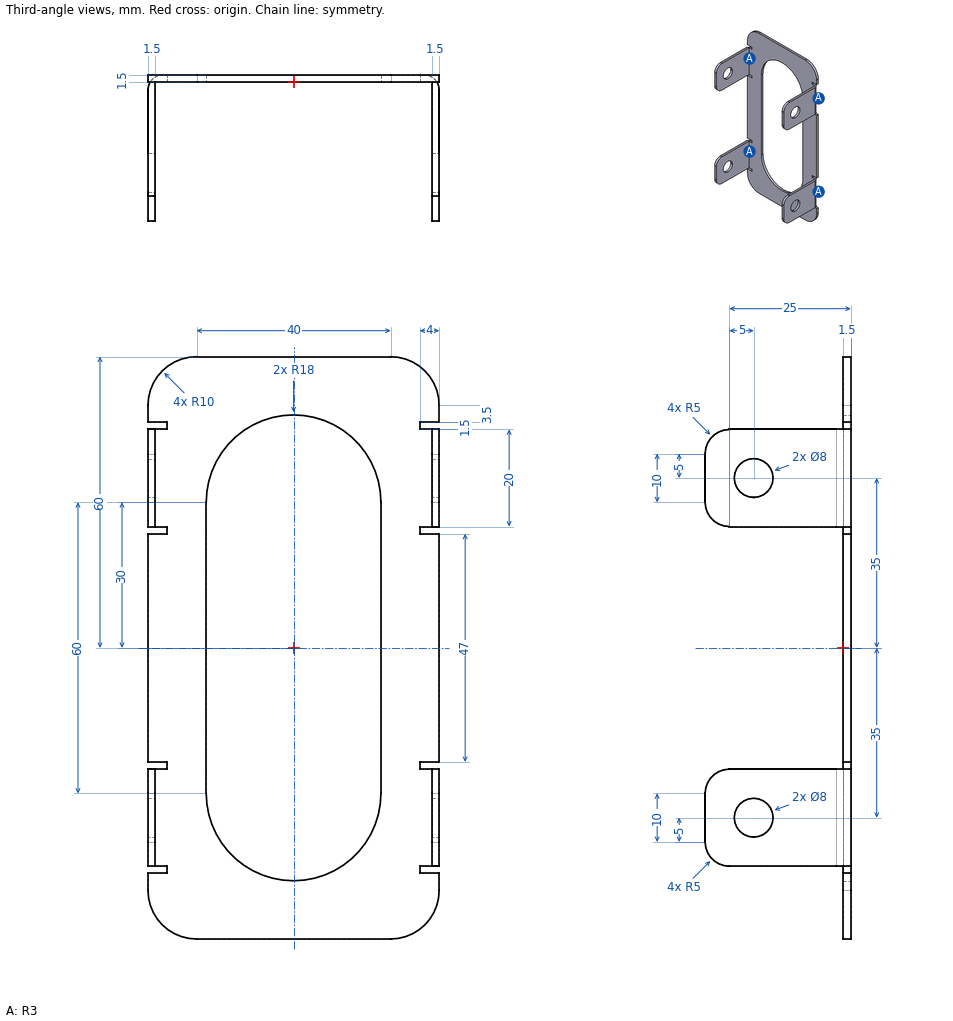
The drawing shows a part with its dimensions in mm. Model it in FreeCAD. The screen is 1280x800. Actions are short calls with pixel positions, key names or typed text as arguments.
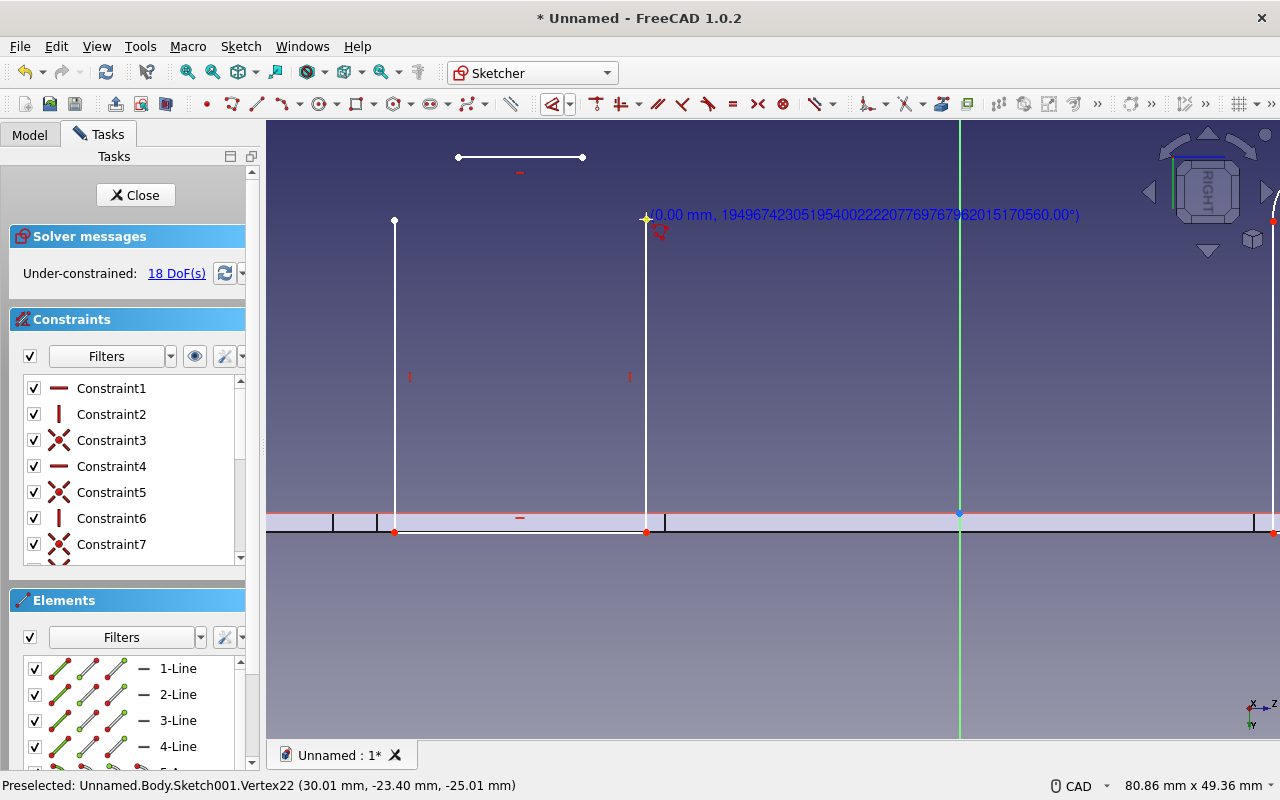
click(282, 104)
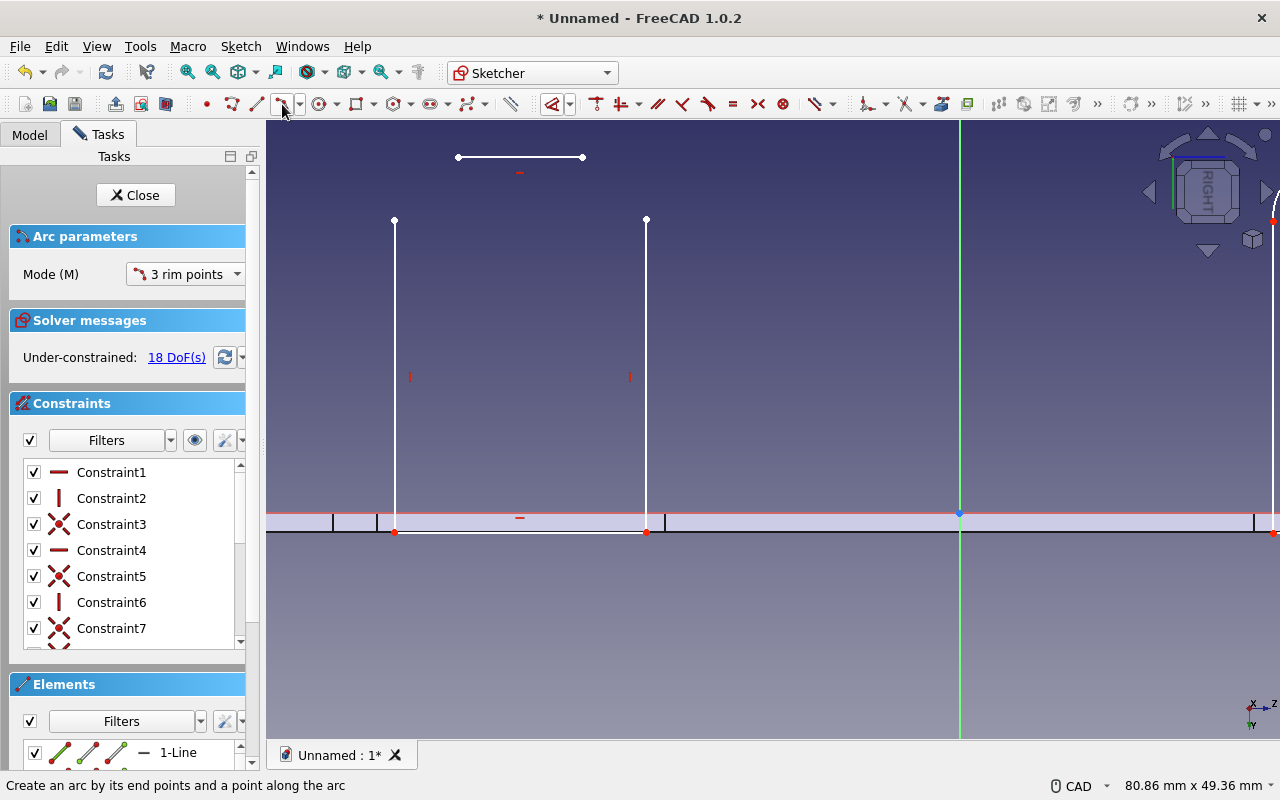
click(459, 157)
click(395, 221)
click(414, 174)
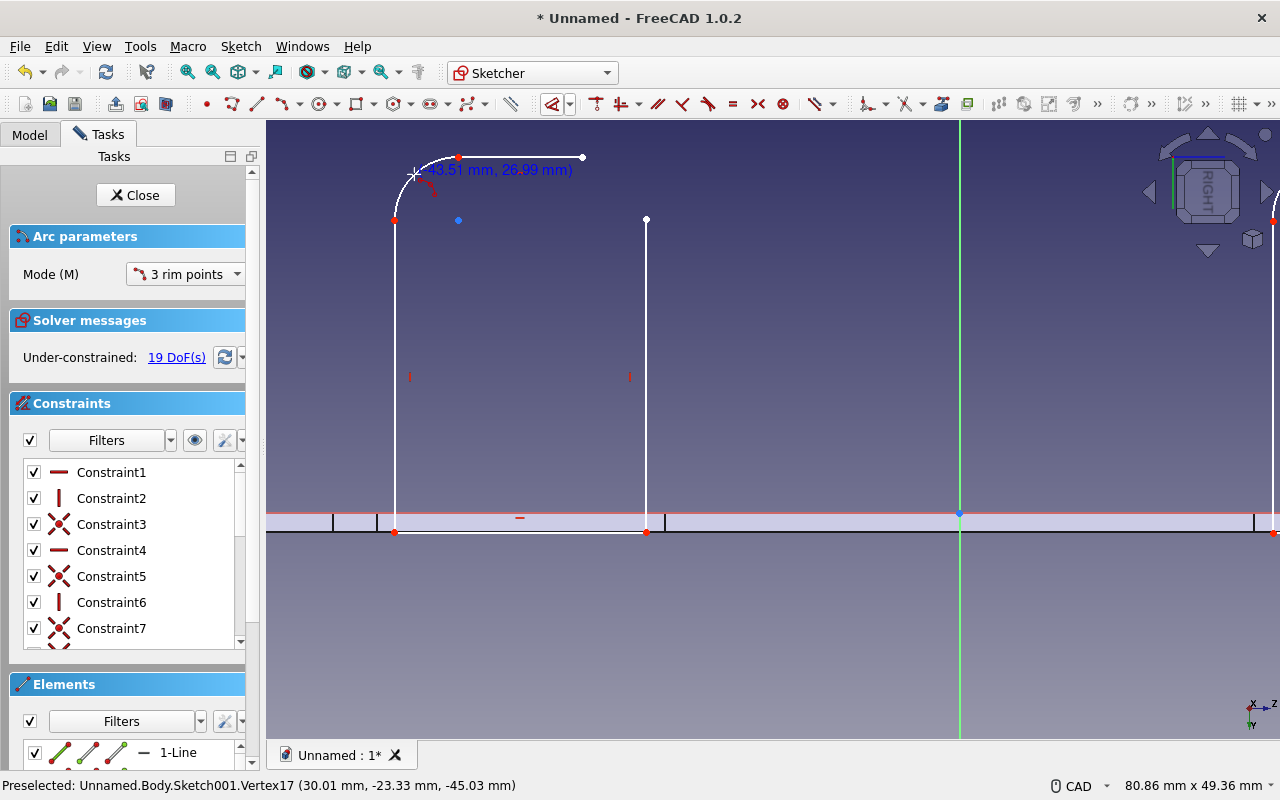
click(646, 220)
click(583, 157)
click(628, 174)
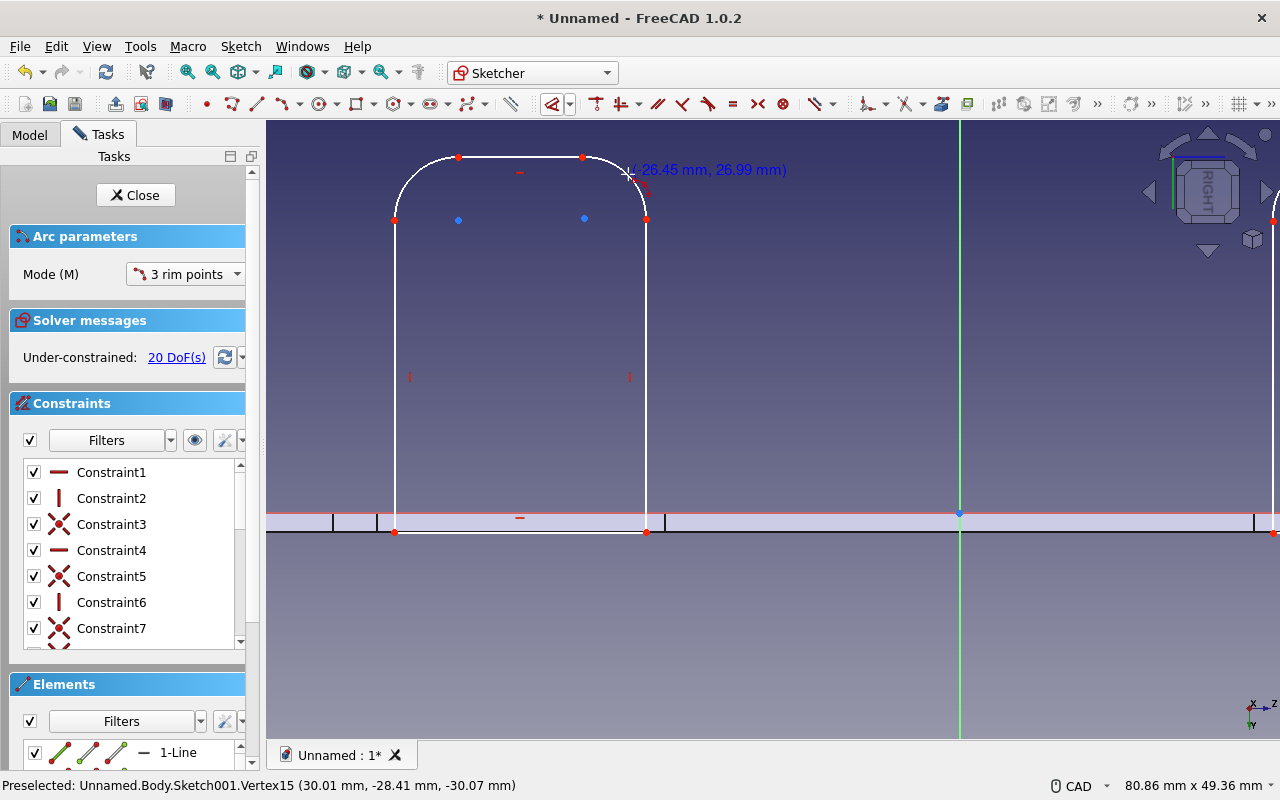
click(318, 104)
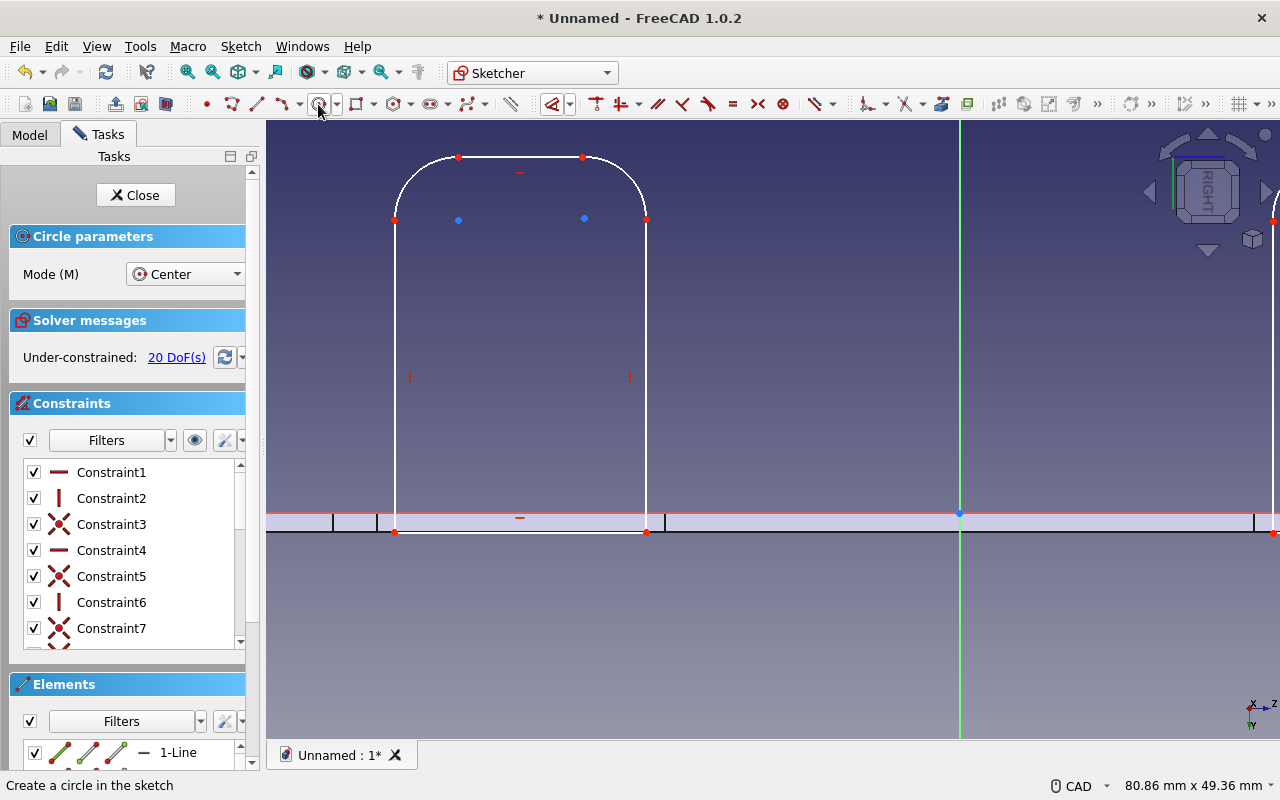
scroll(394, 533, down, 3)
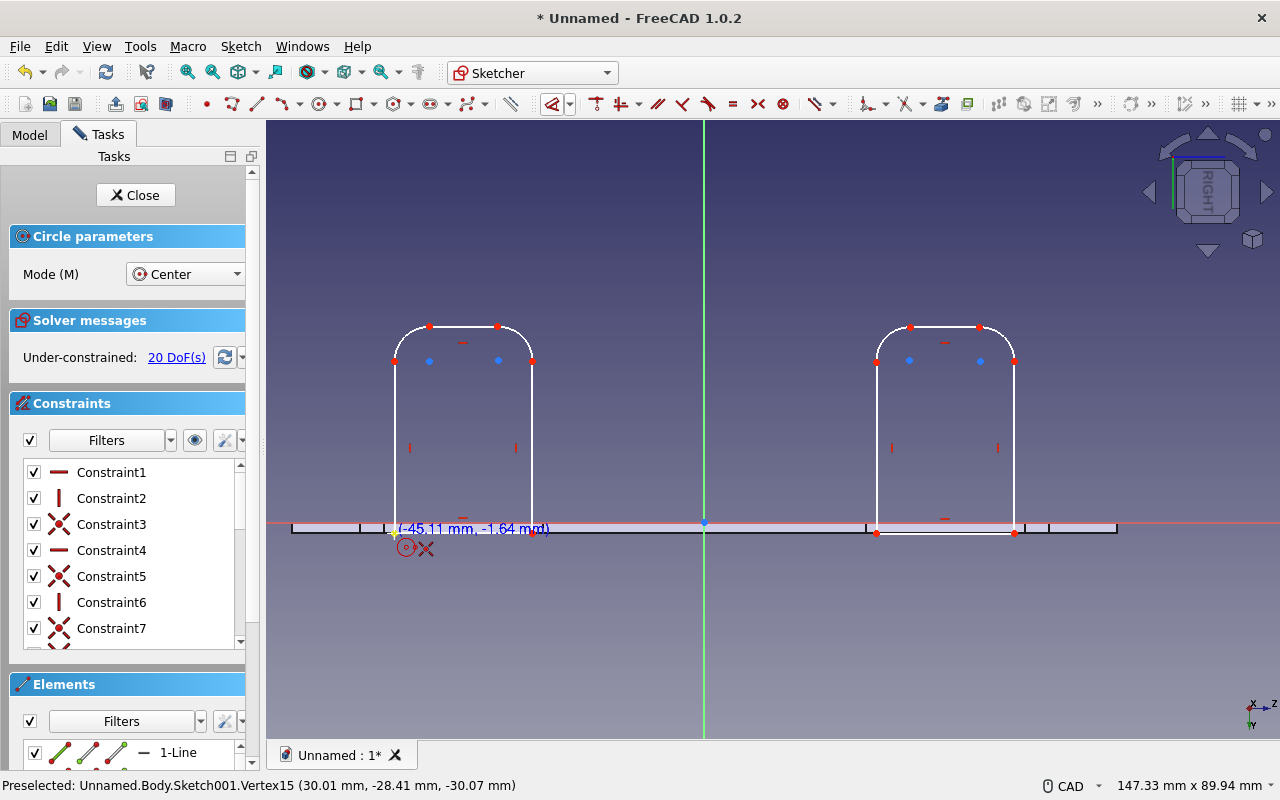
click(945, 395)
move(965, 376)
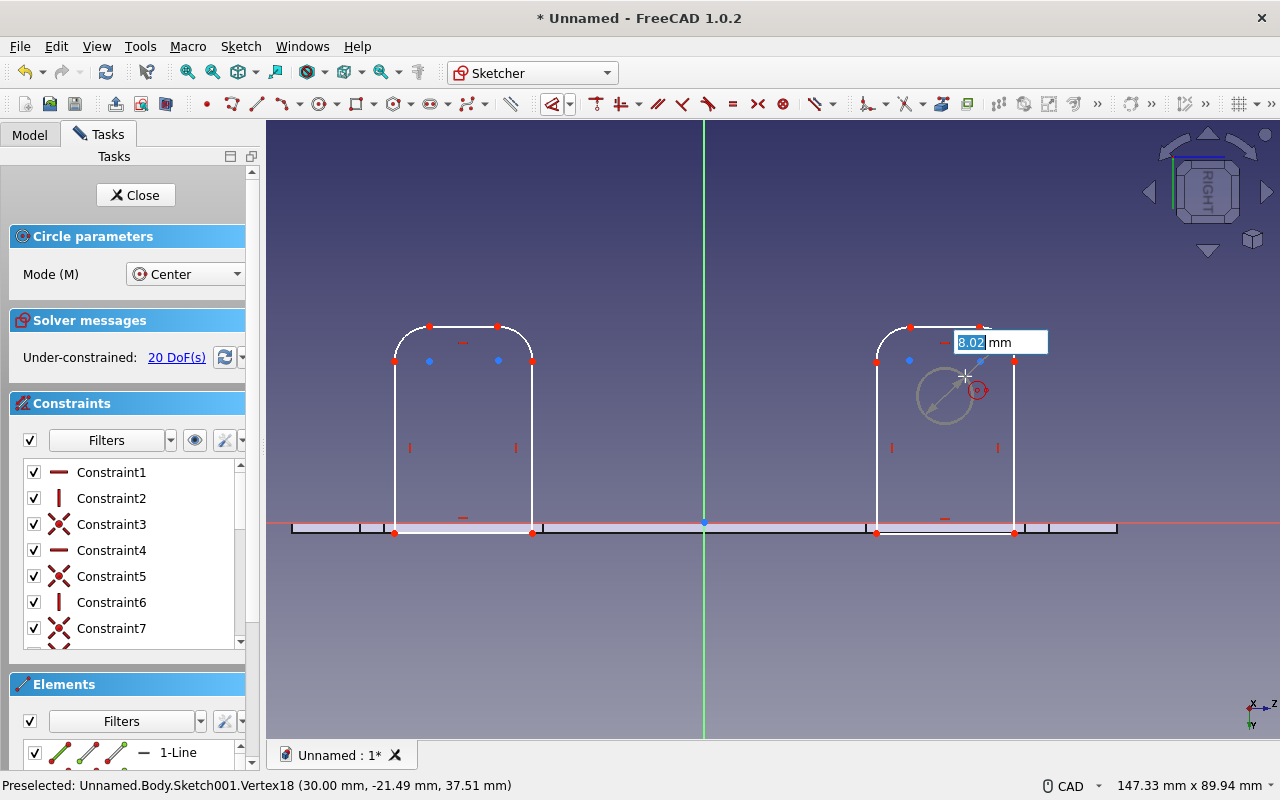
text(8)
key(Return)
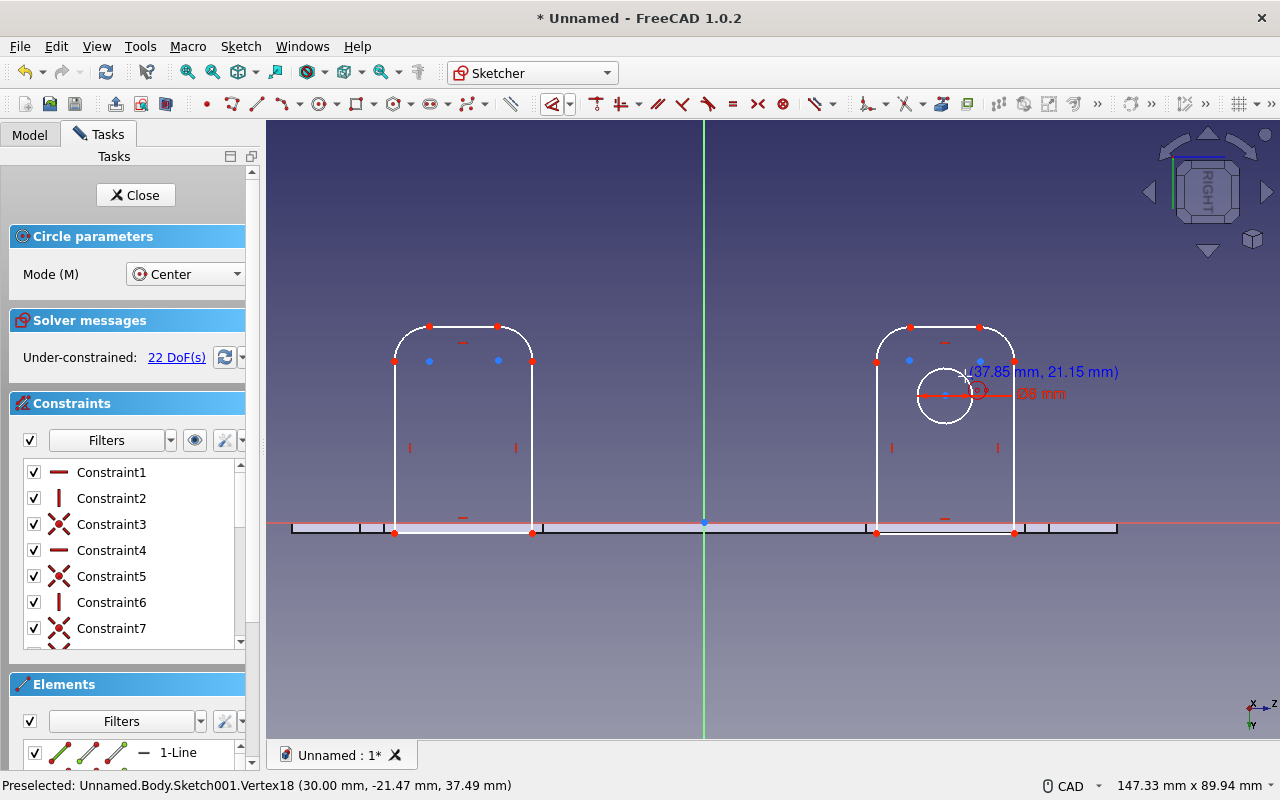
click(464, 395)
move(483, 376)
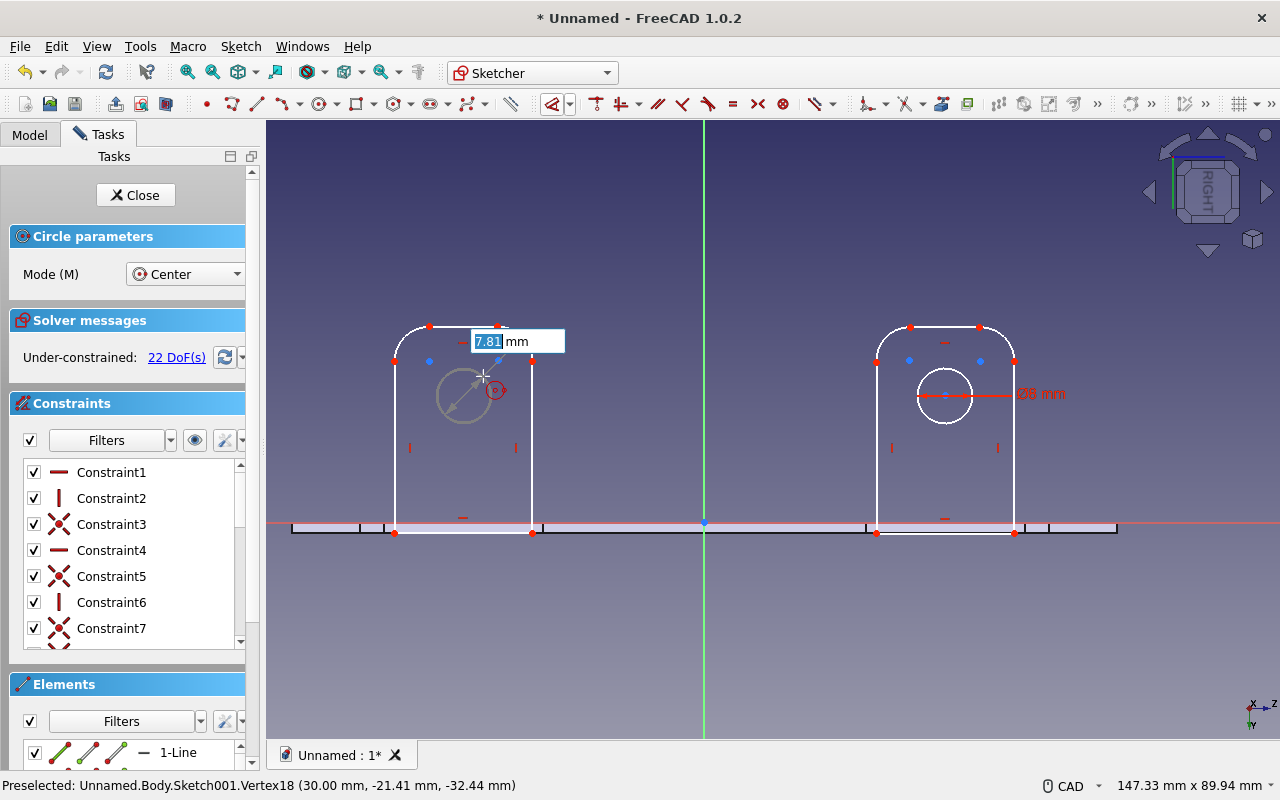
text(8)
key(Return)
key(Escape)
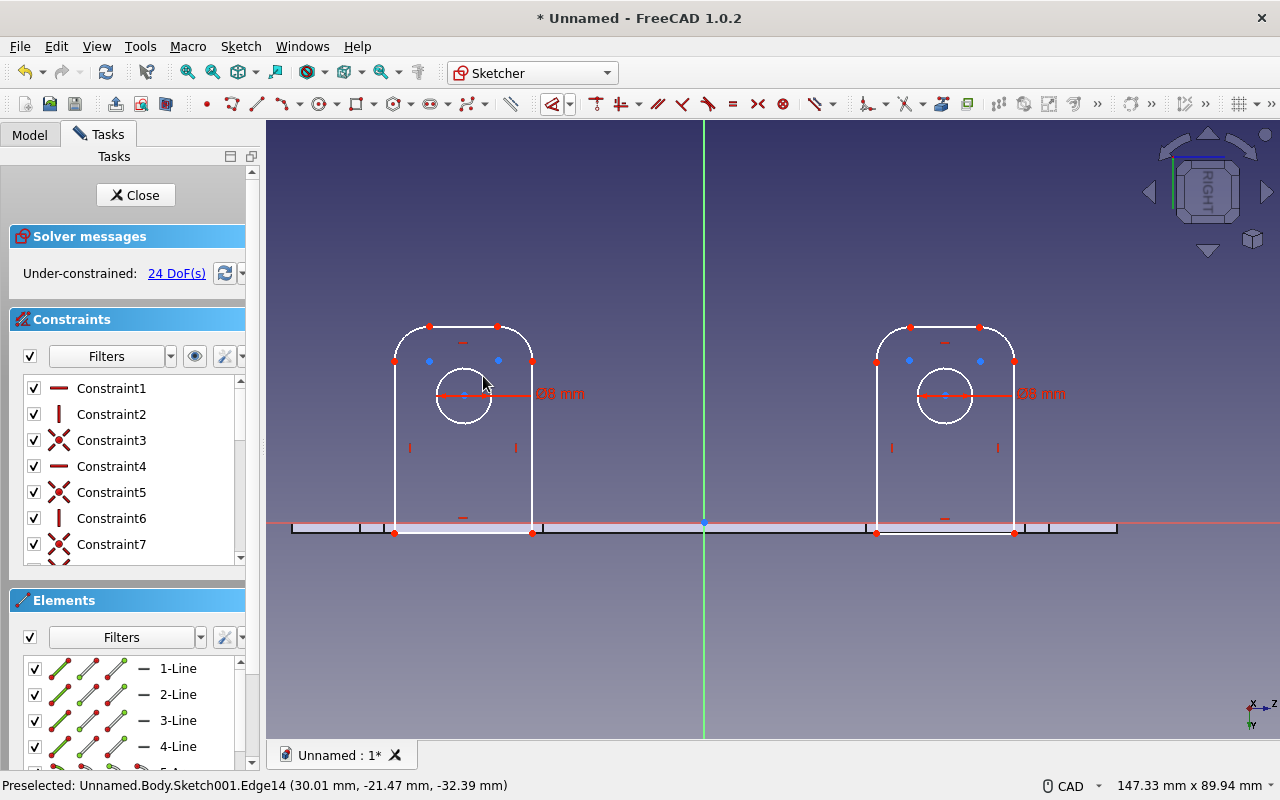
click(959, 327)